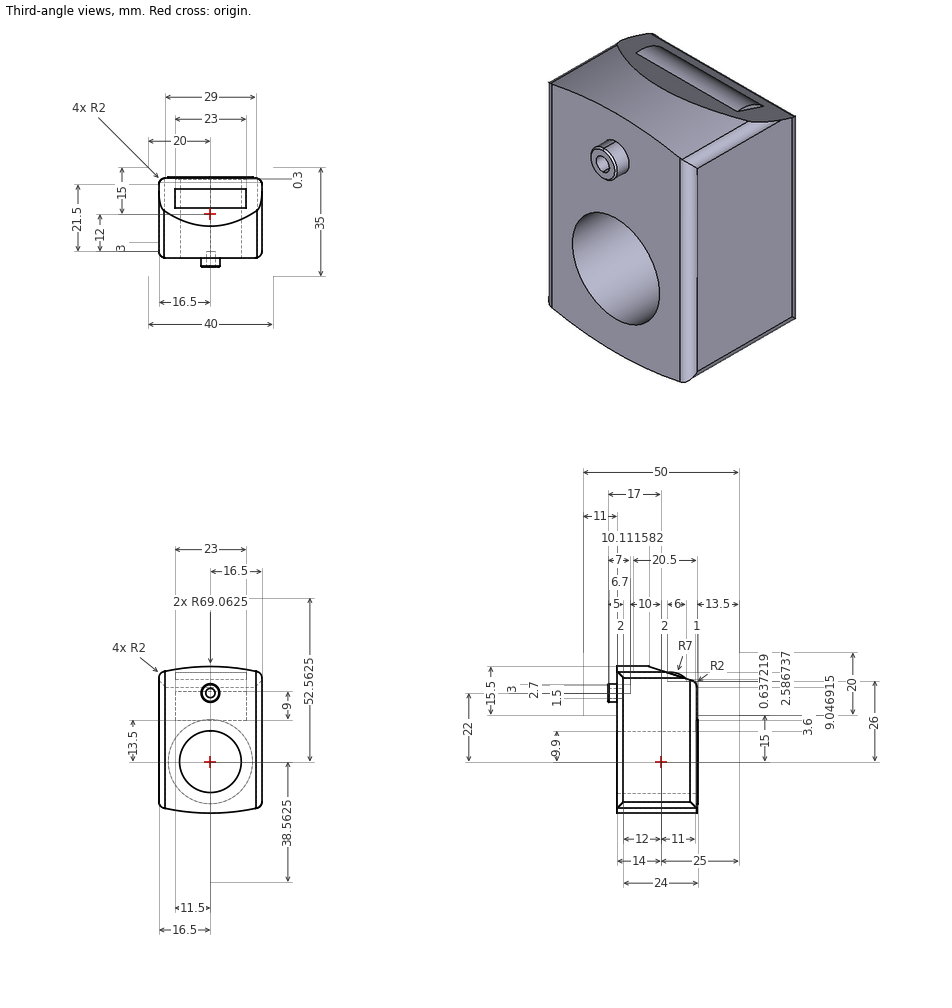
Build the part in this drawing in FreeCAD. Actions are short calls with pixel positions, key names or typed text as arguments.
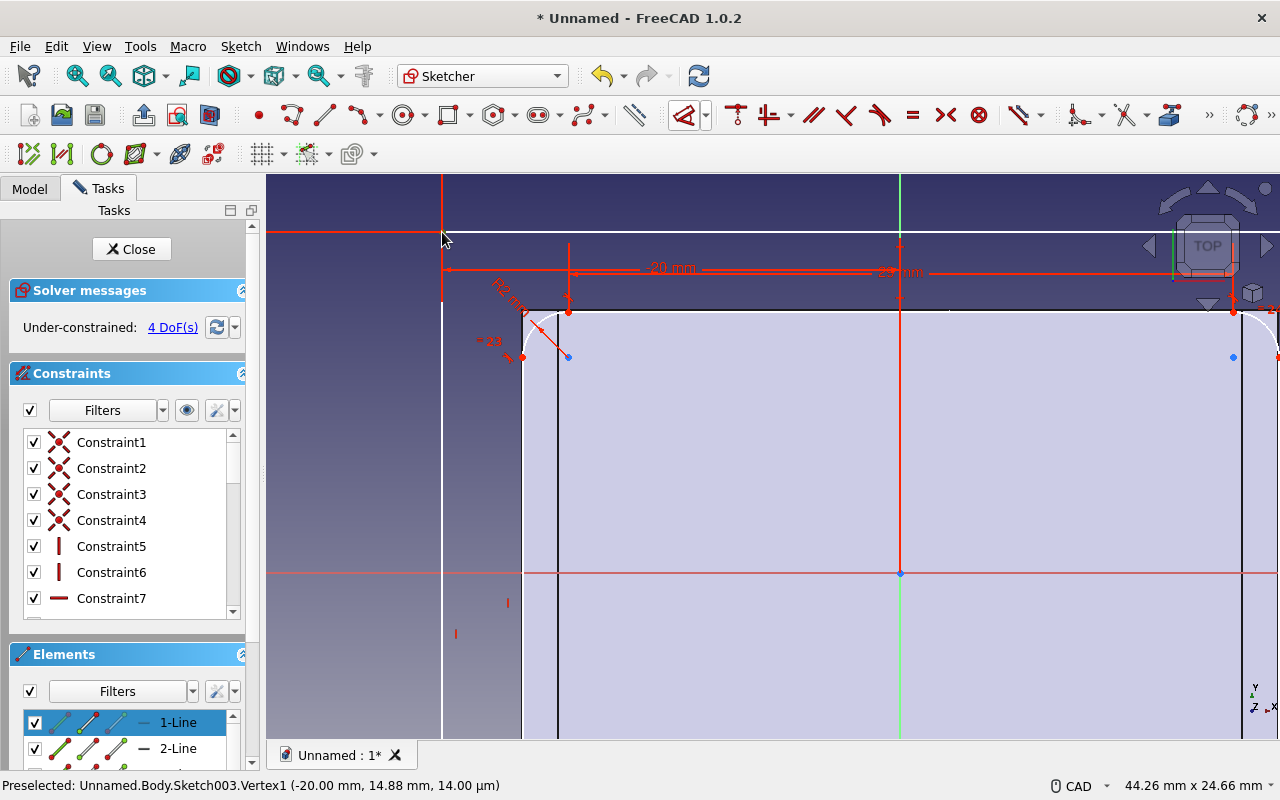
key(i)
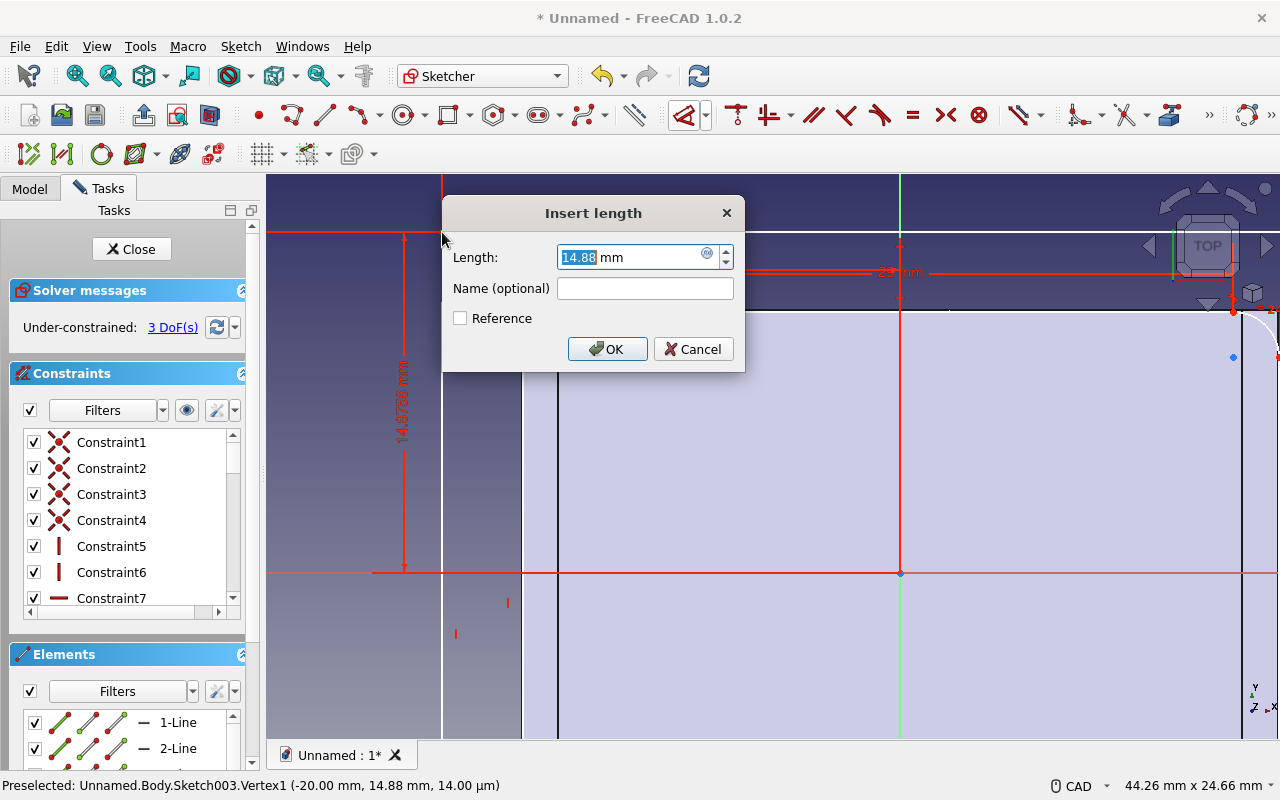
text(15)
key(Return)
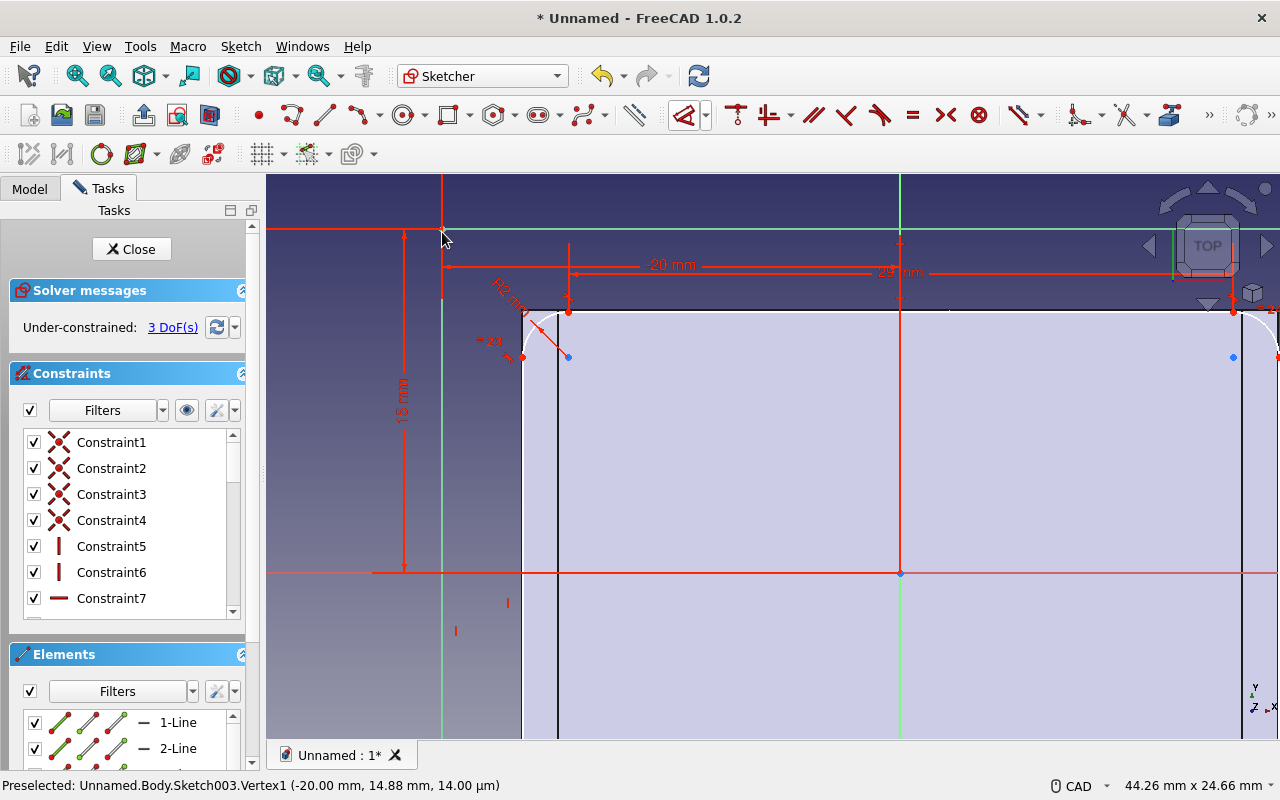
scroll(545, 315, down, 4)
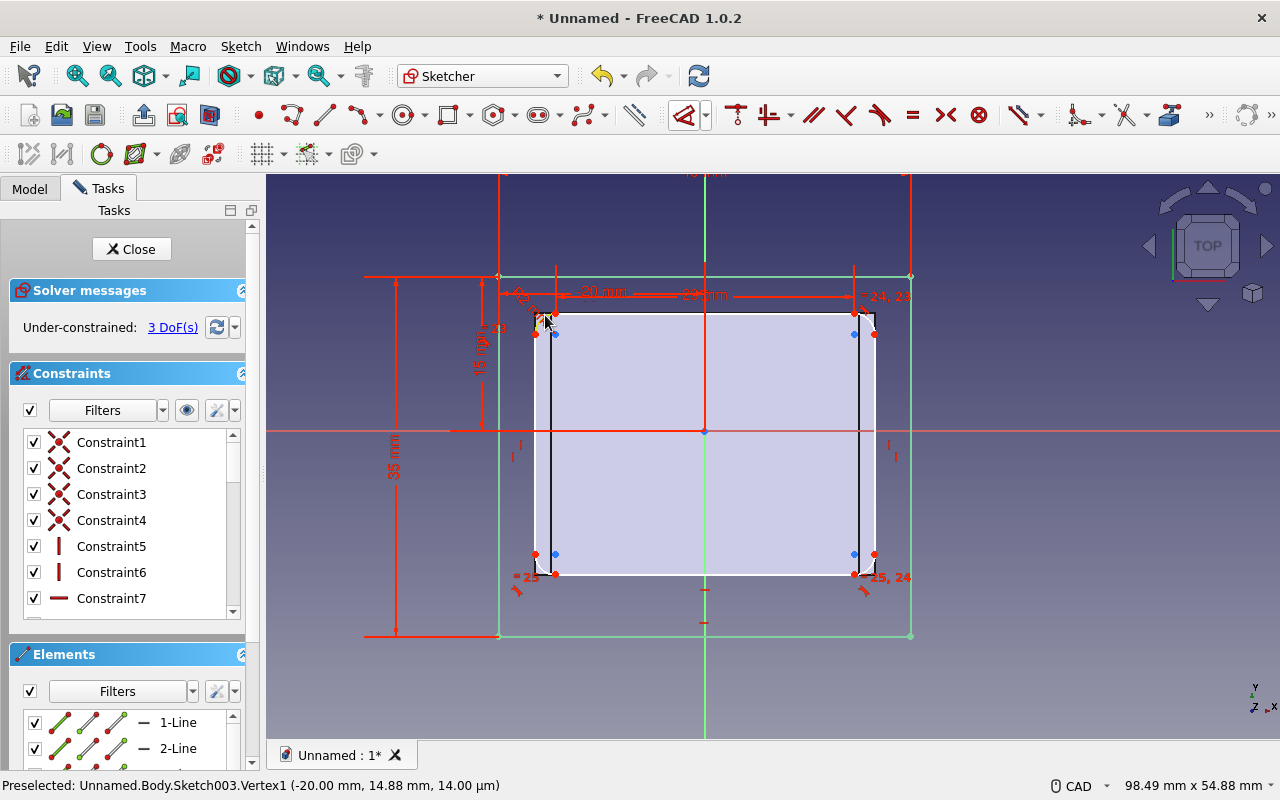
click(535, 554)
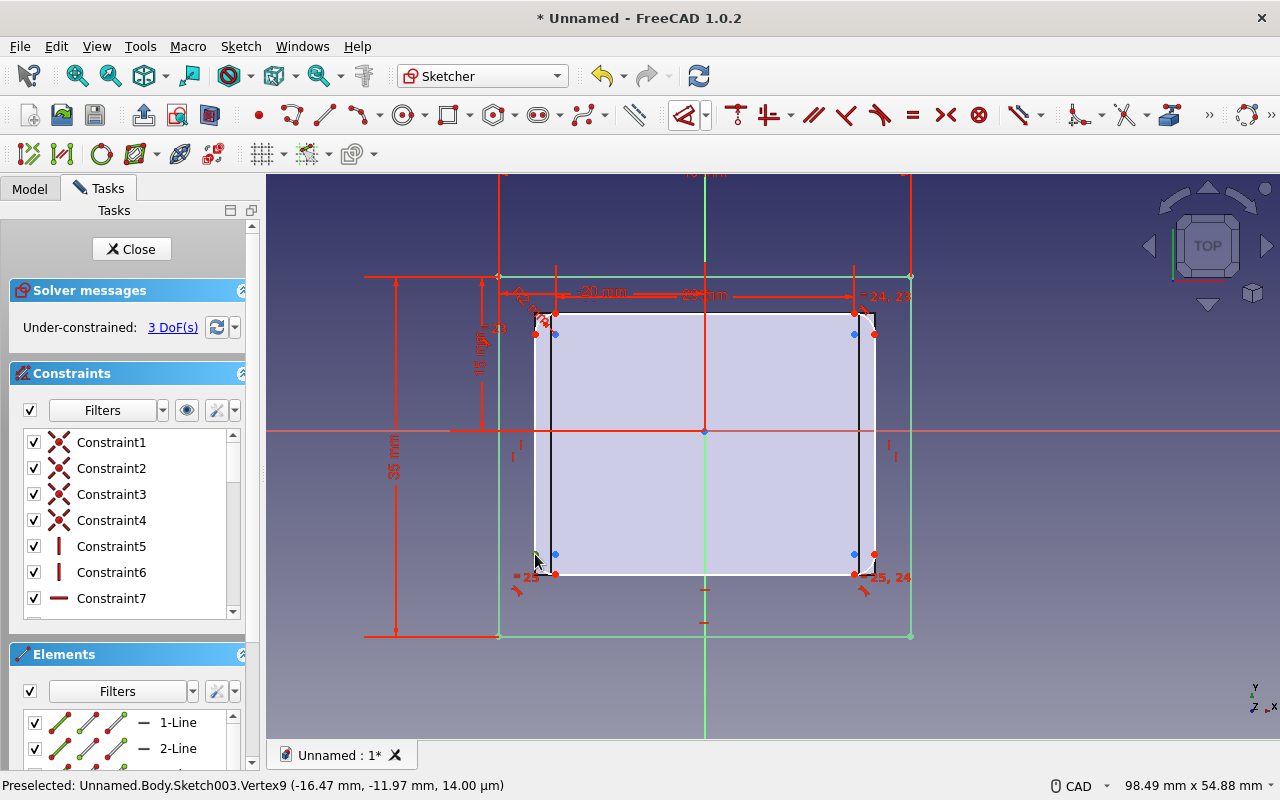
click(706, 116)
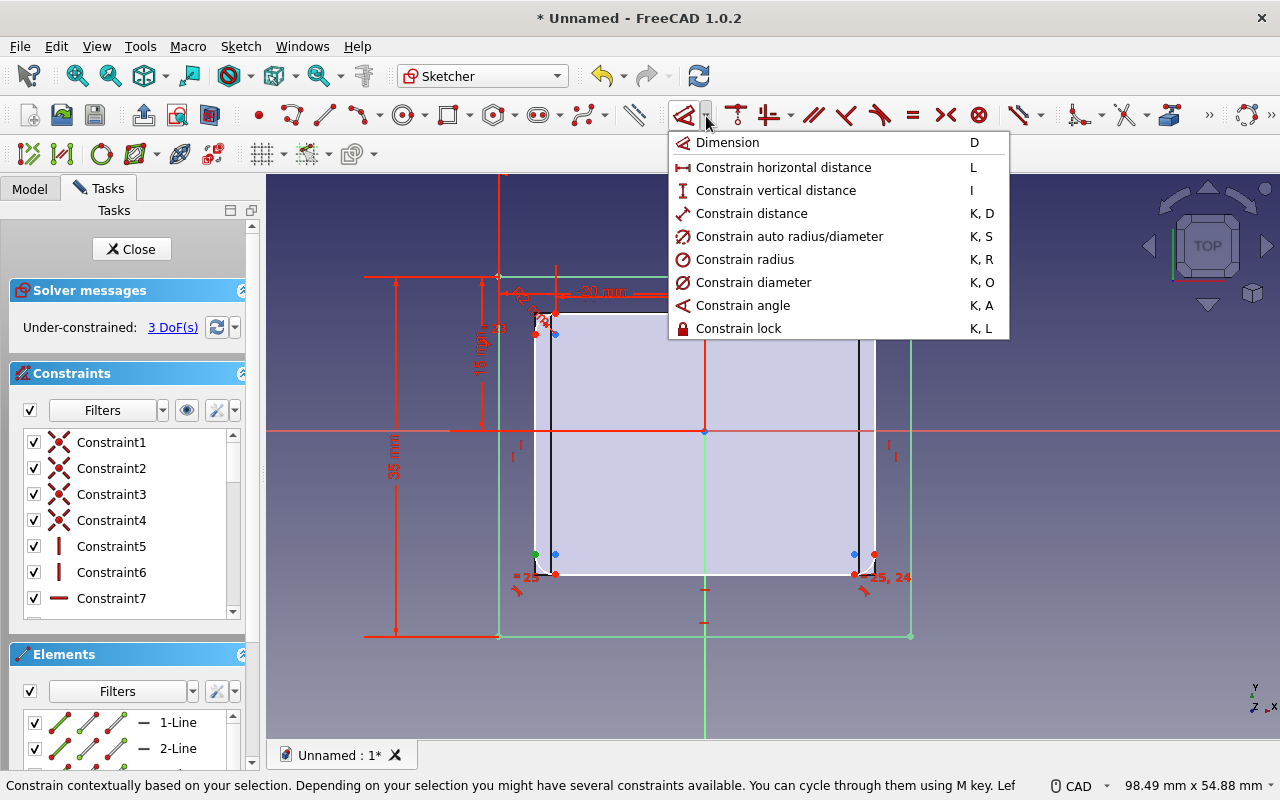
click(839, 190)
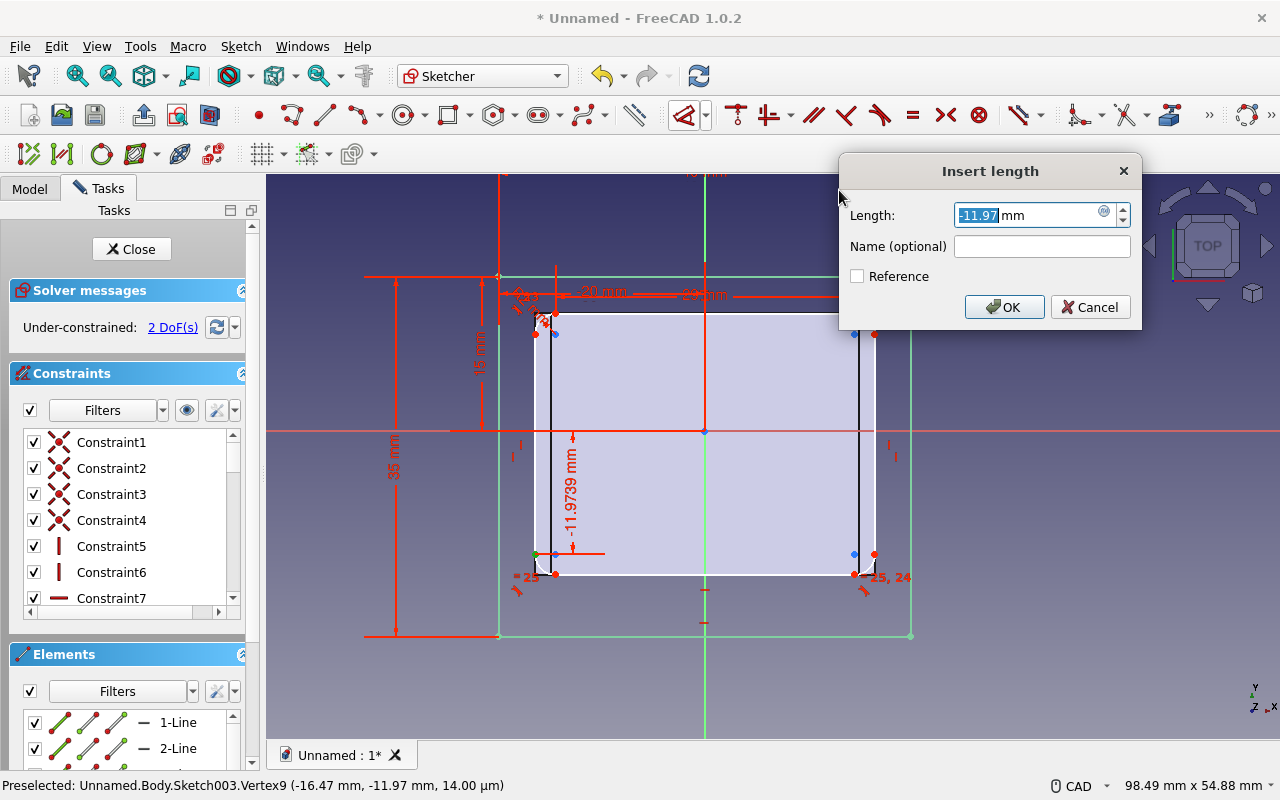
text(-12)
key(Return)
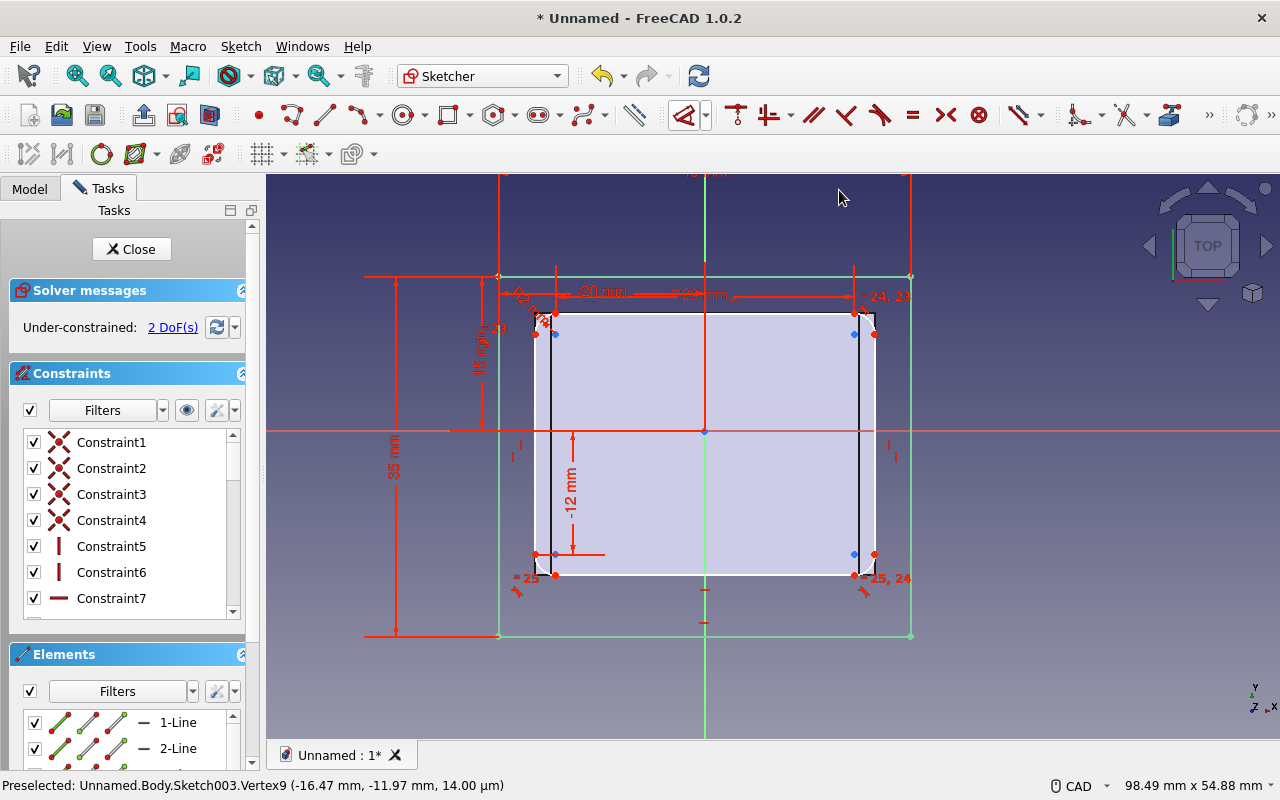
click(535, 489)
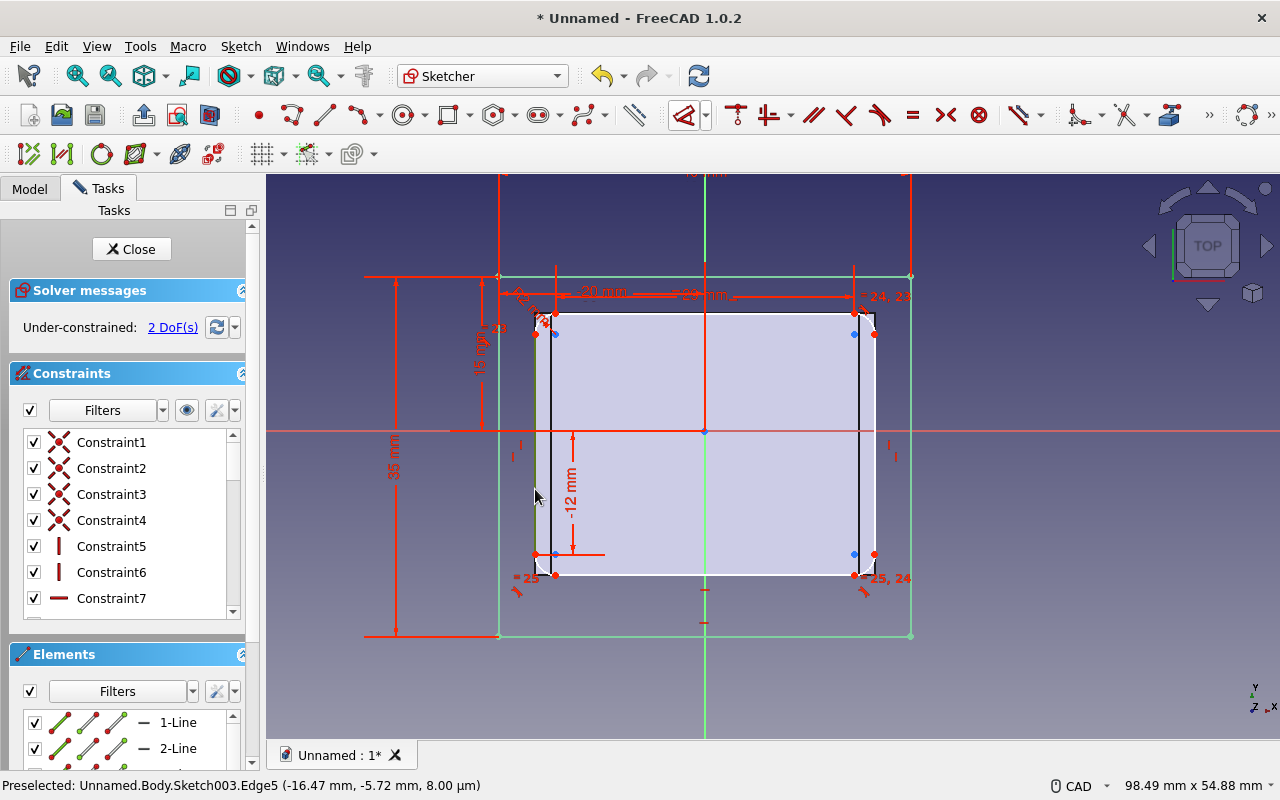
key(i)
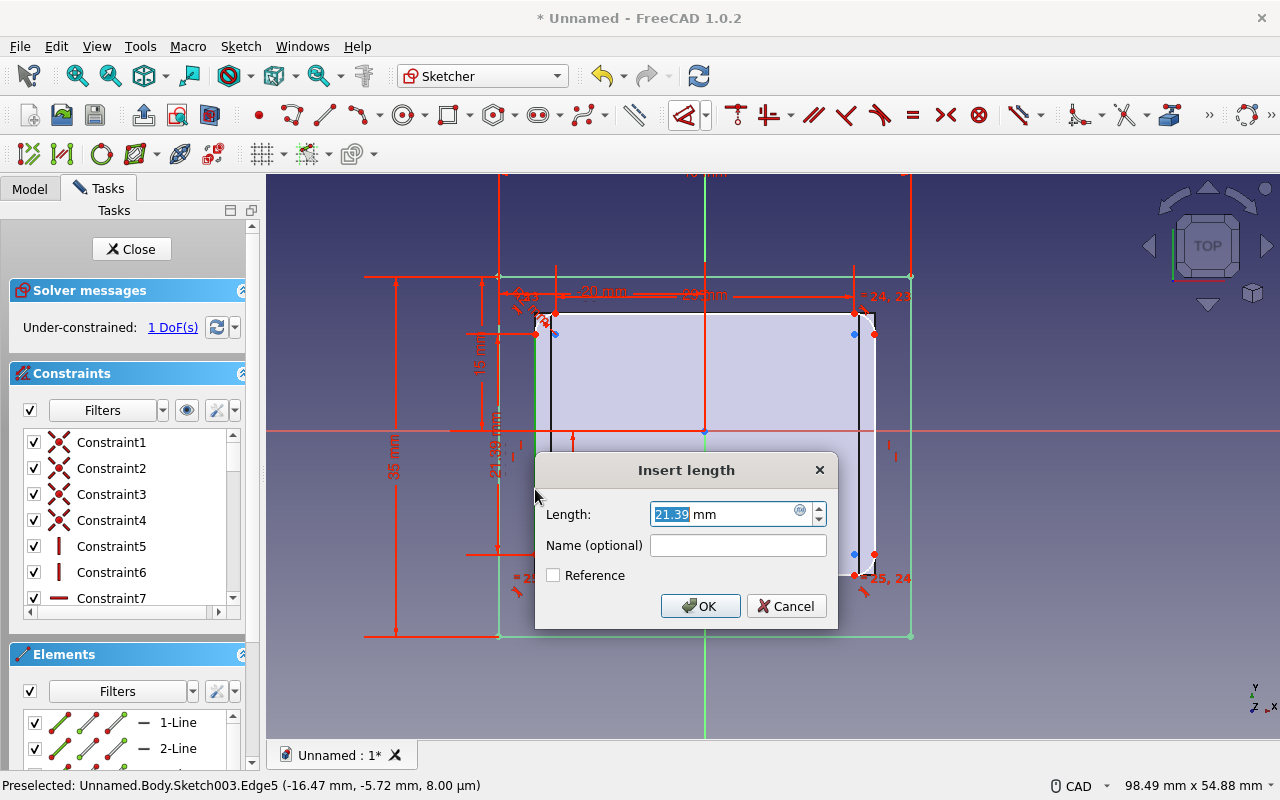
text(21.5)
key(Return)